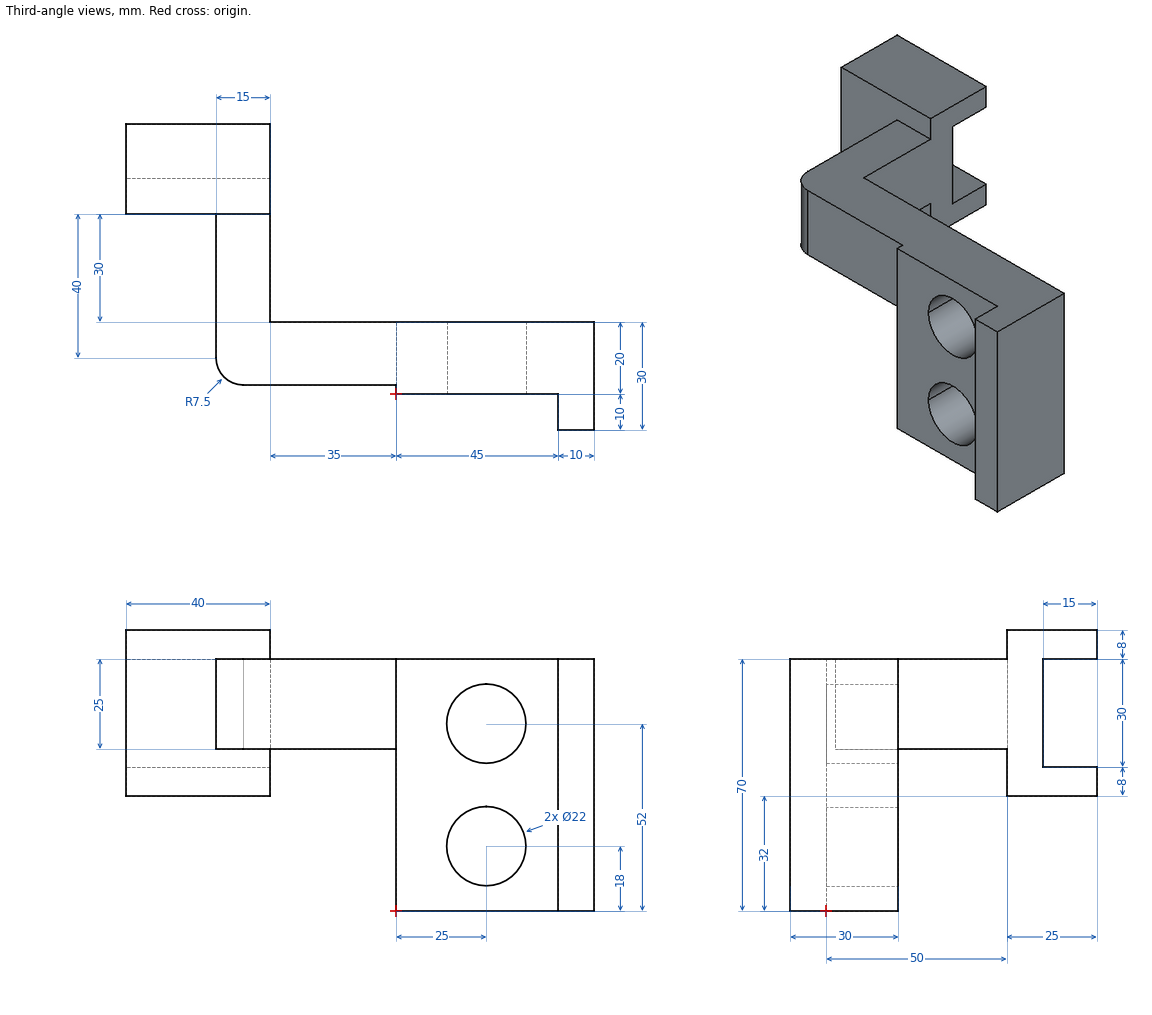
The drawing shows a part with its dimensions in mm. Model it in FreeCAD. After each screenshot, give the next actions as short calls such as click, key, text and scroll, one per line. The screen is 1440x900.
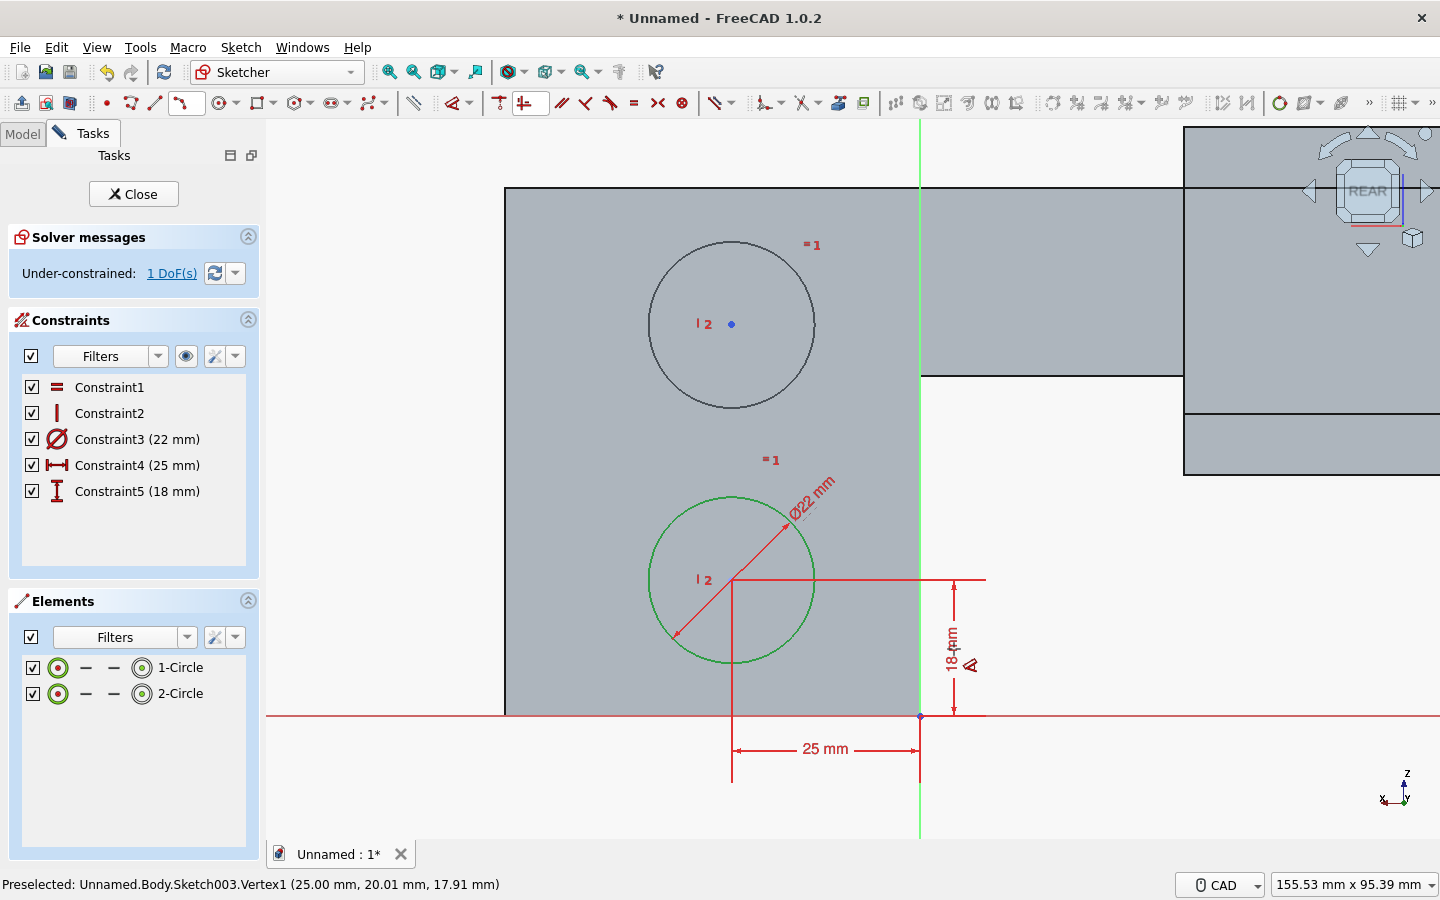
click(732, 325)
click(954, 521)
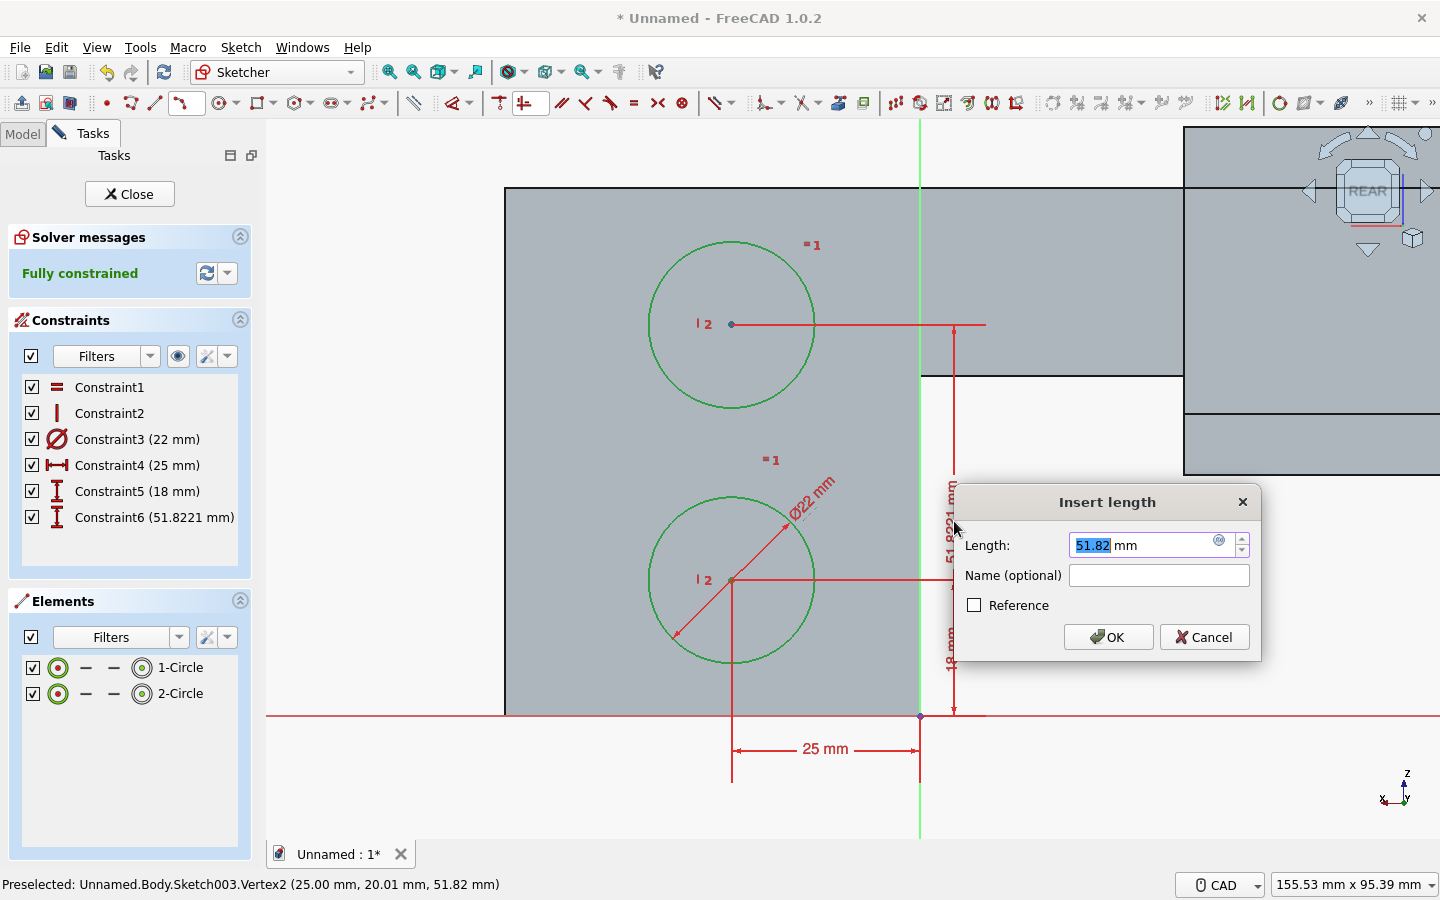
text(52)
key(Return)
key(Escape)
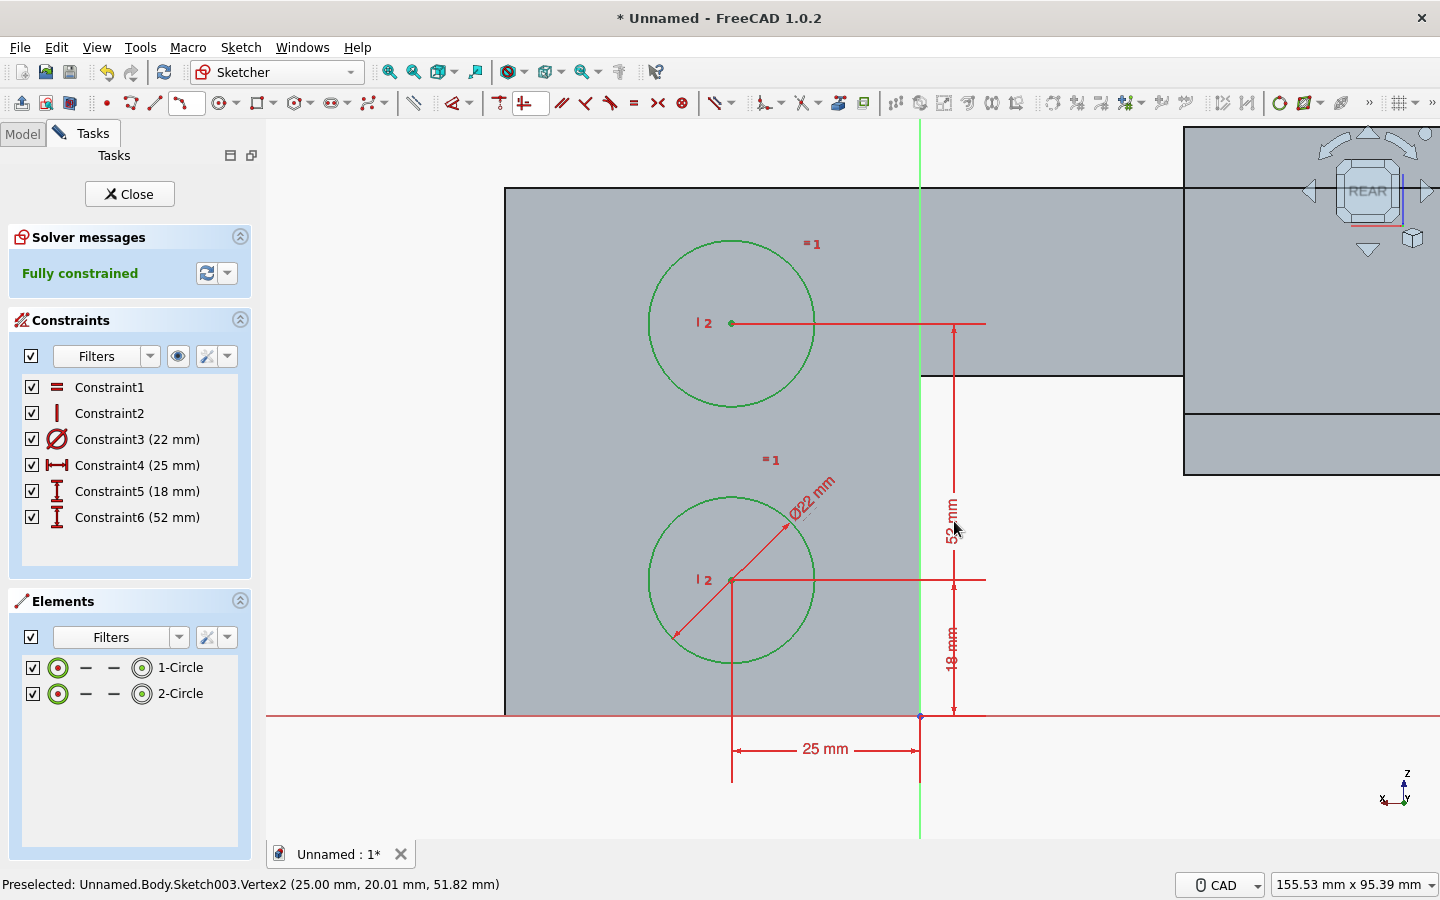
click(130, 194)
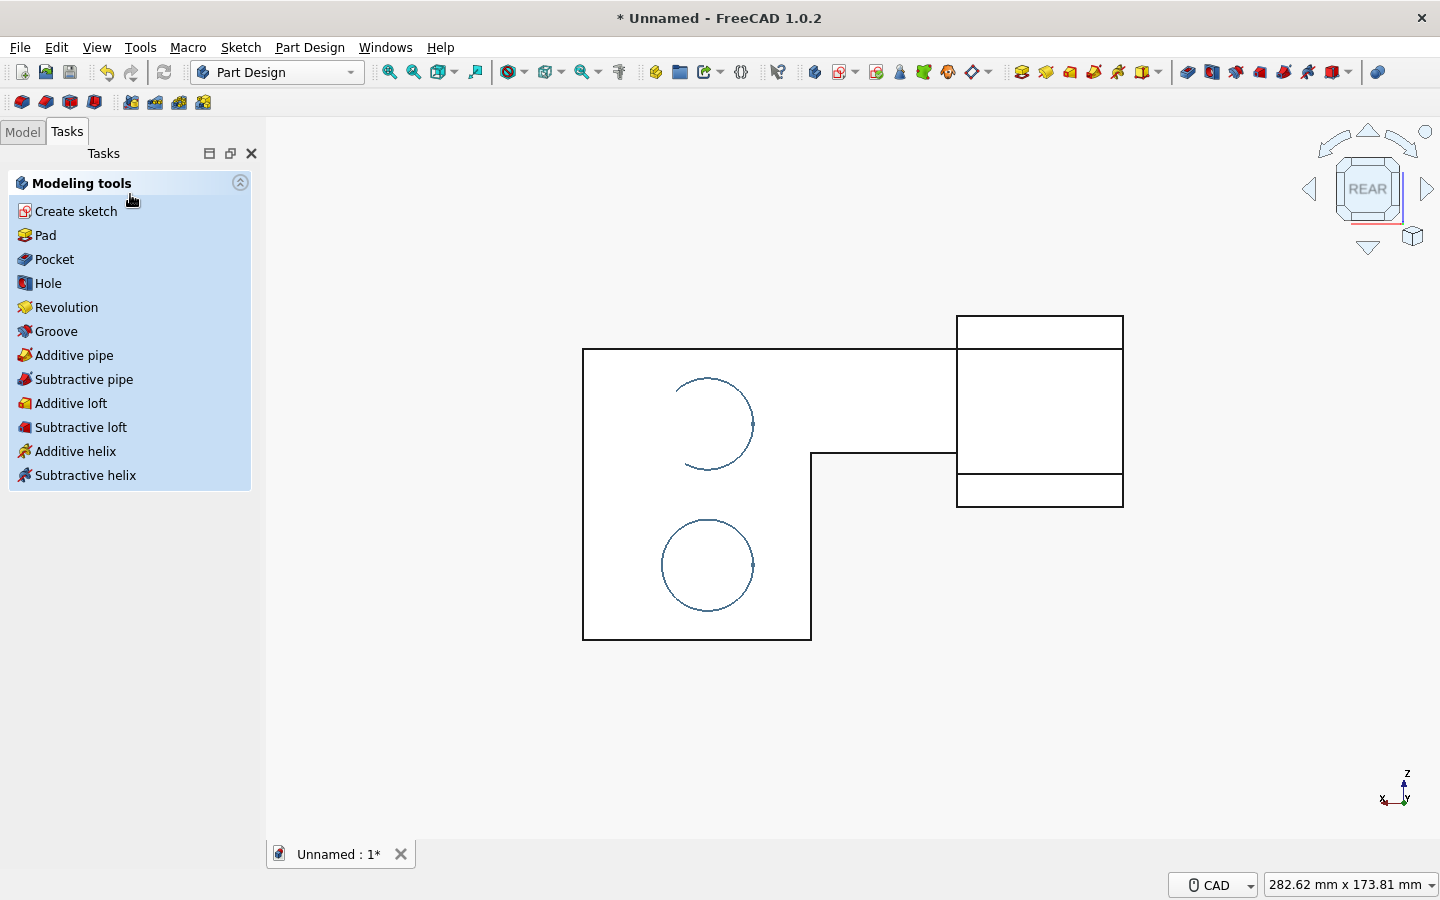
click(1188, 72)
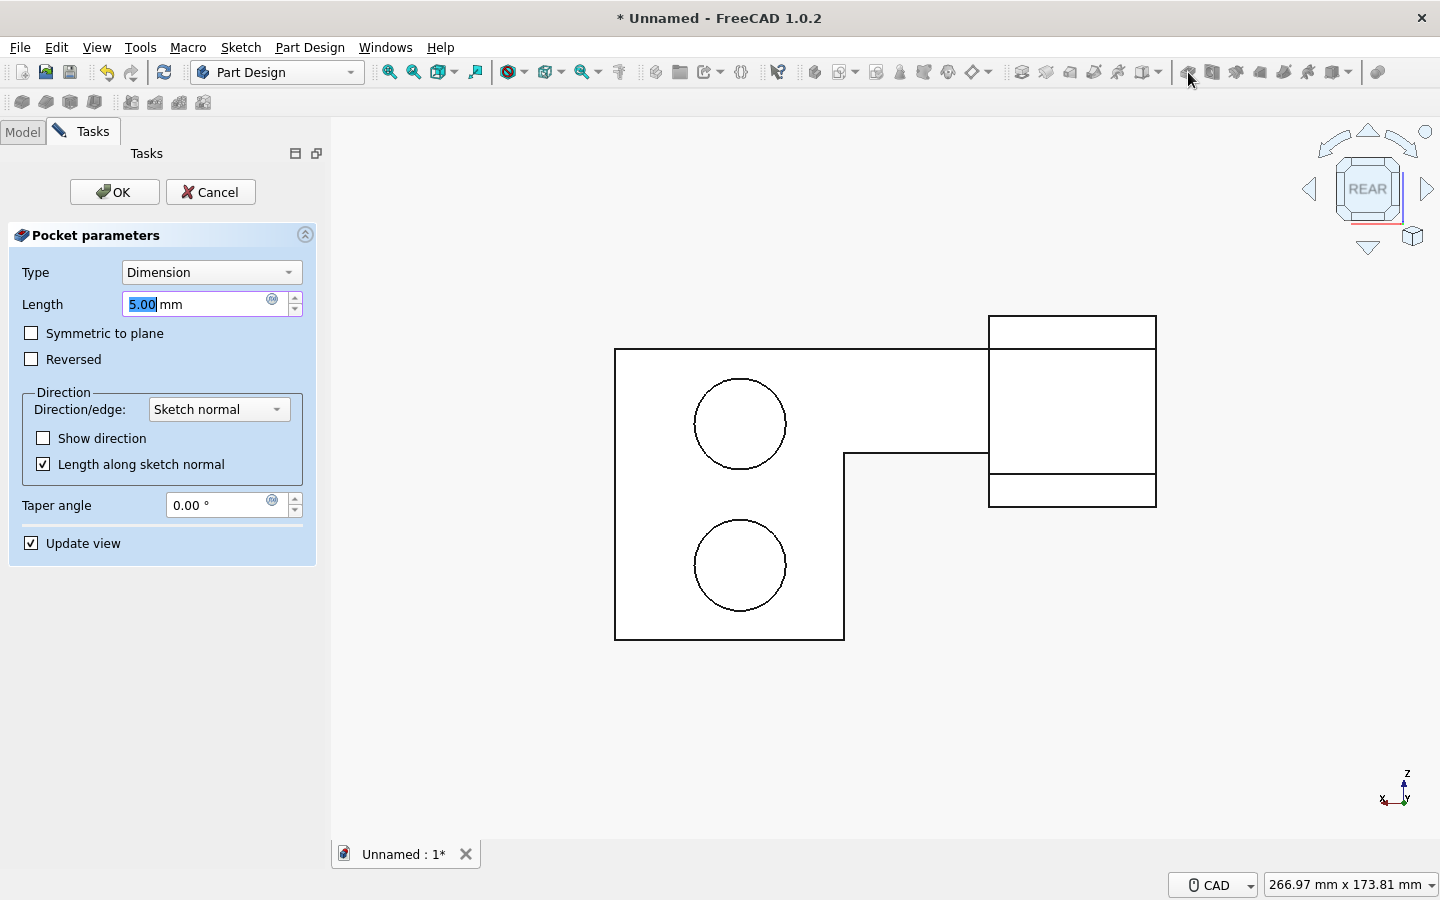
text(30)
key(Tab)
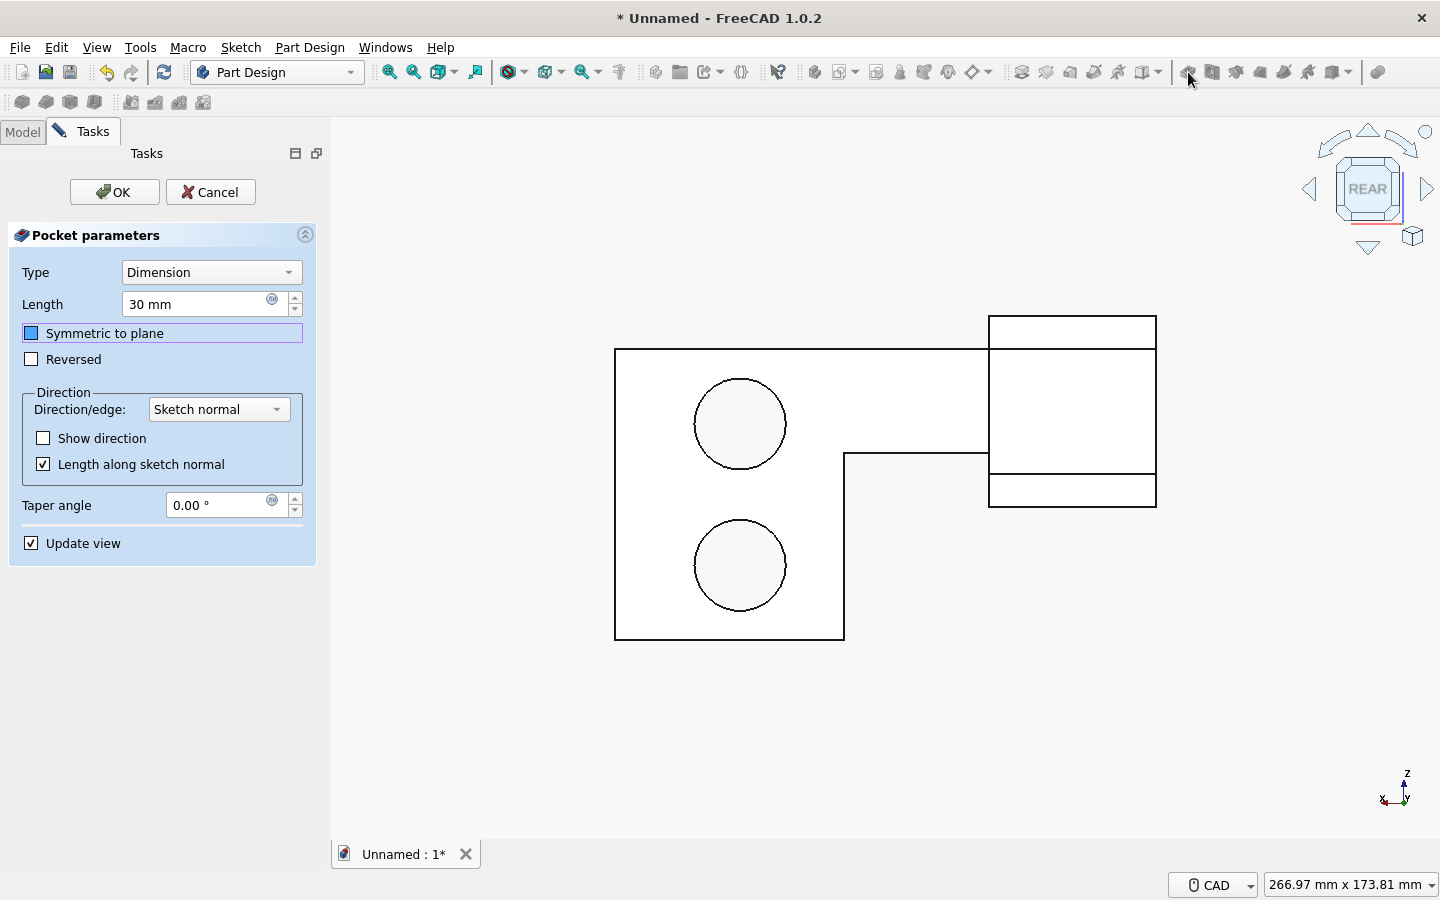
click(115, 192)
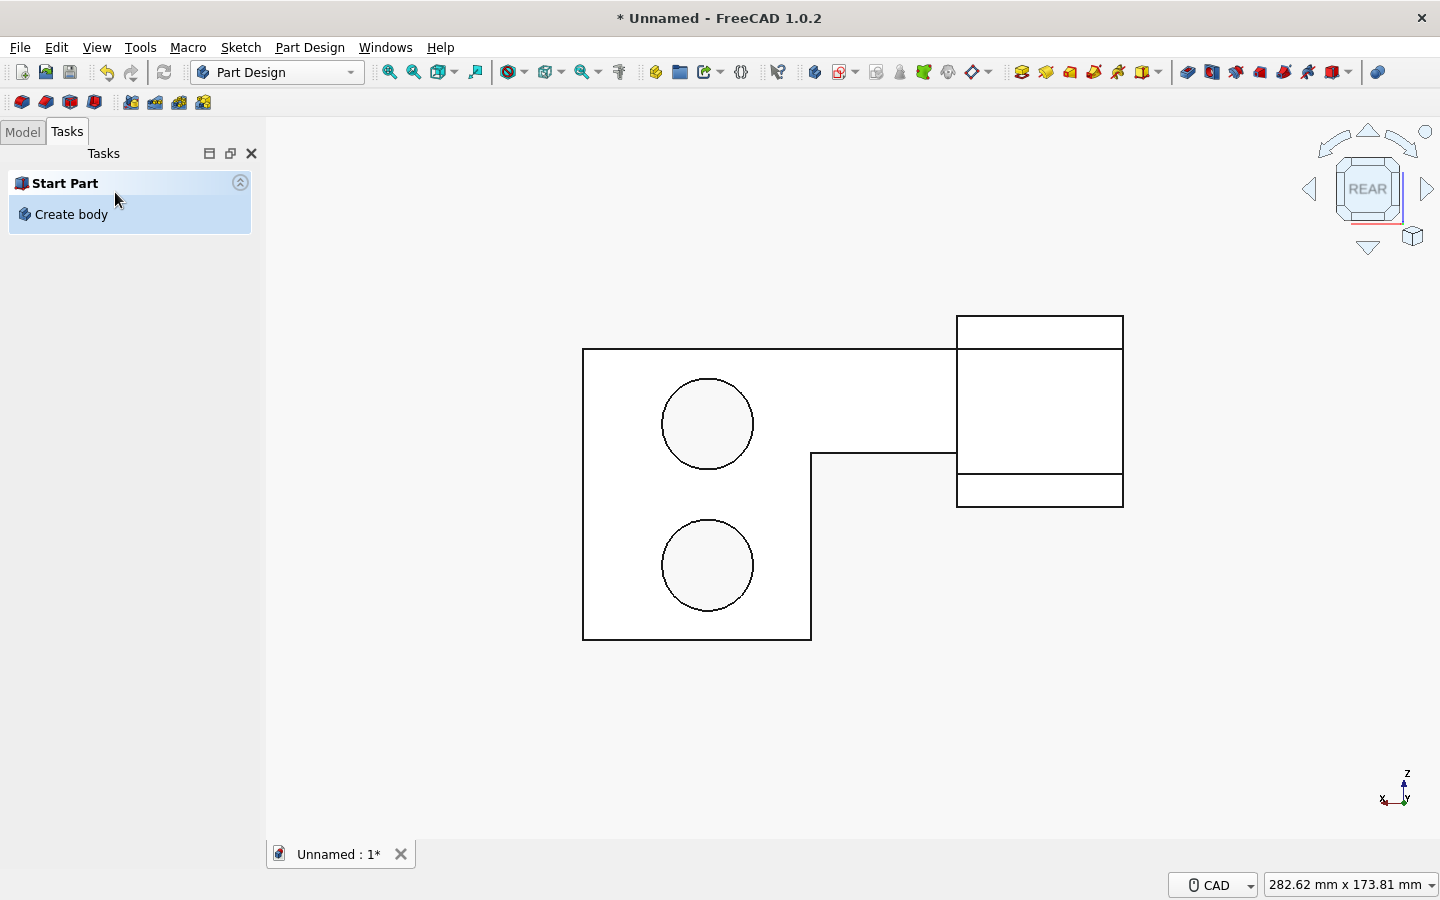
key(0)